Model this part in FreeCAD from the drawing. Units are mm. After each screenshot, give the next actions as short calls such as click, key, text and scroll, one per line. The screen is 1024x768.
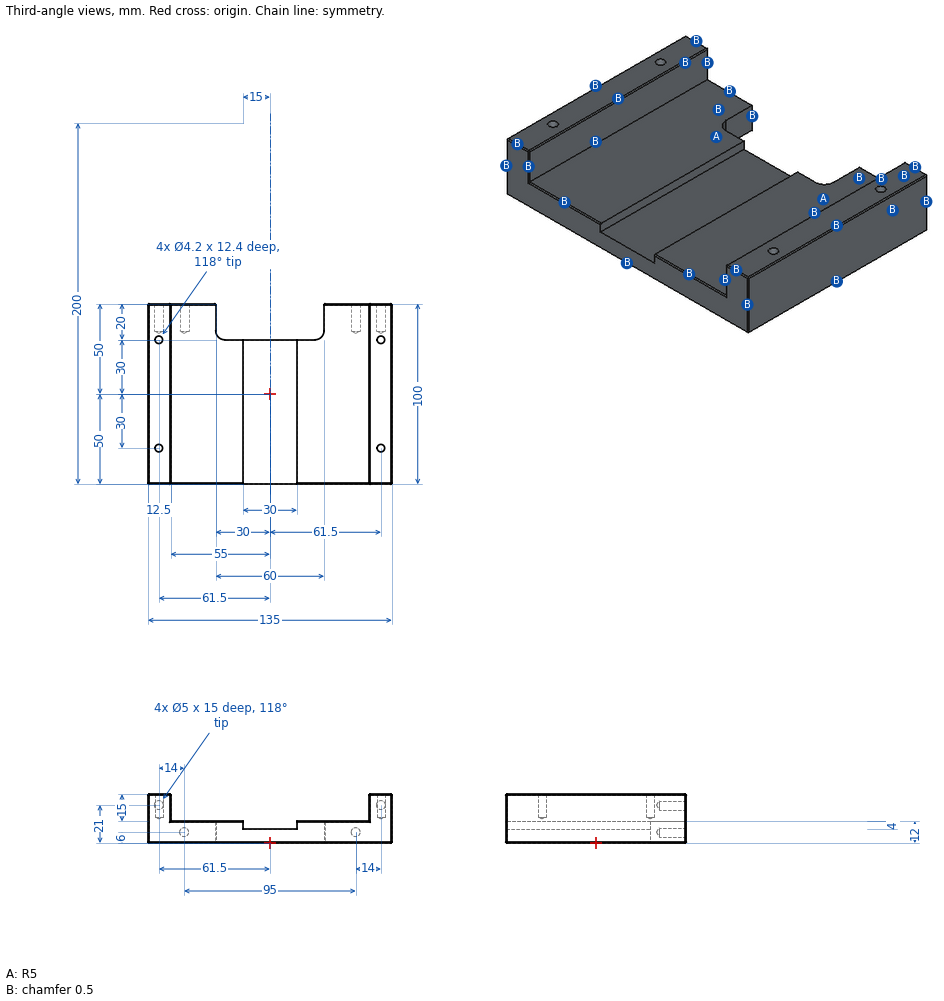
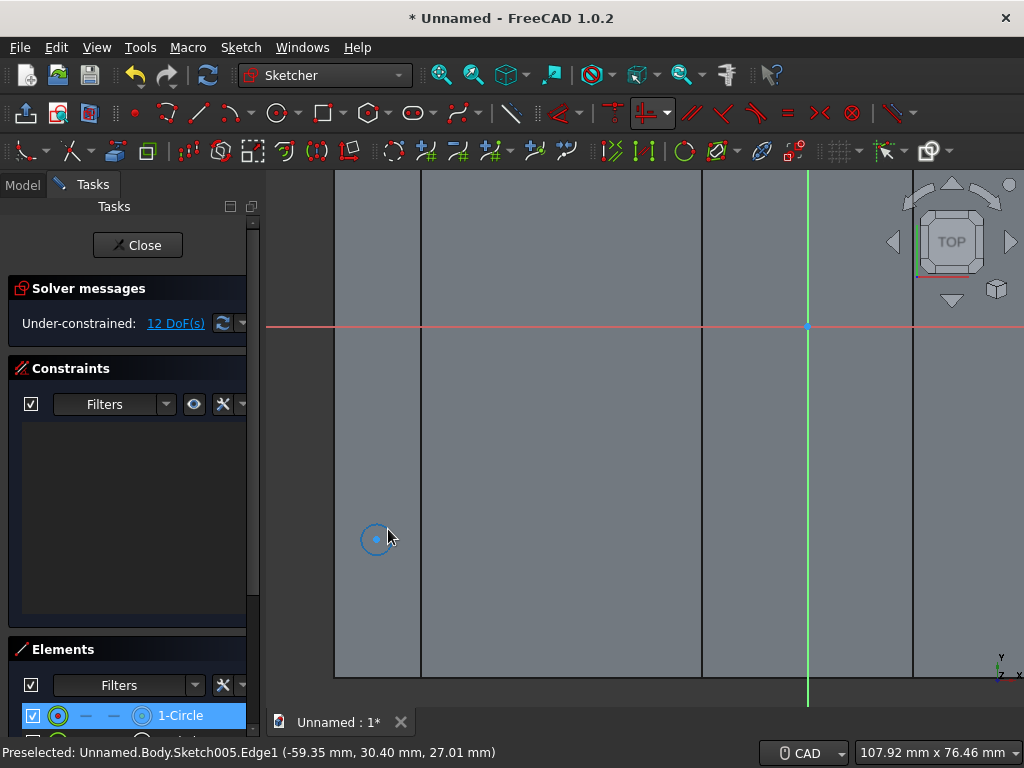
click(388, 529)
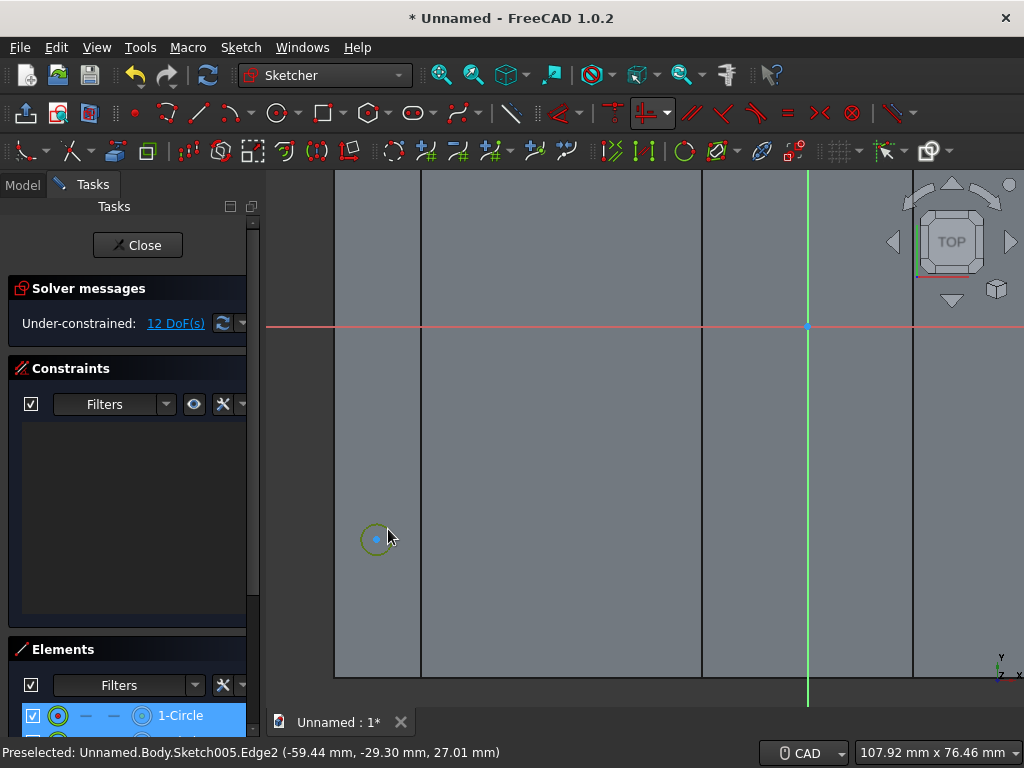
scroll(388, 530, down, 4)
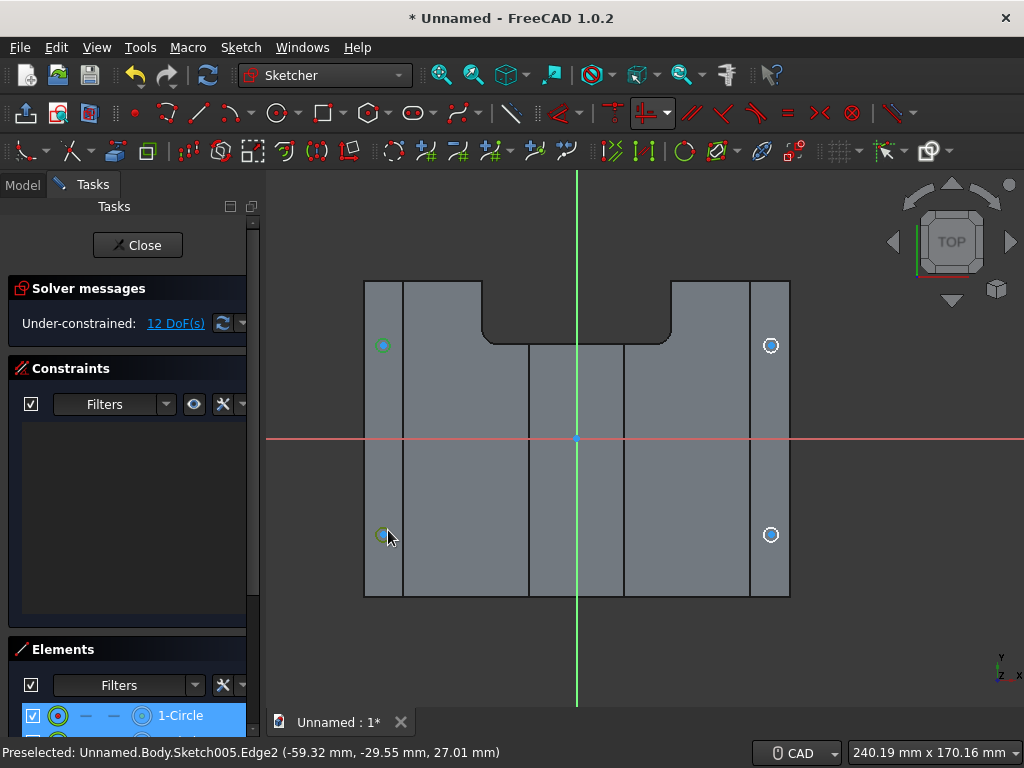
scroll(776, 530, up, 4)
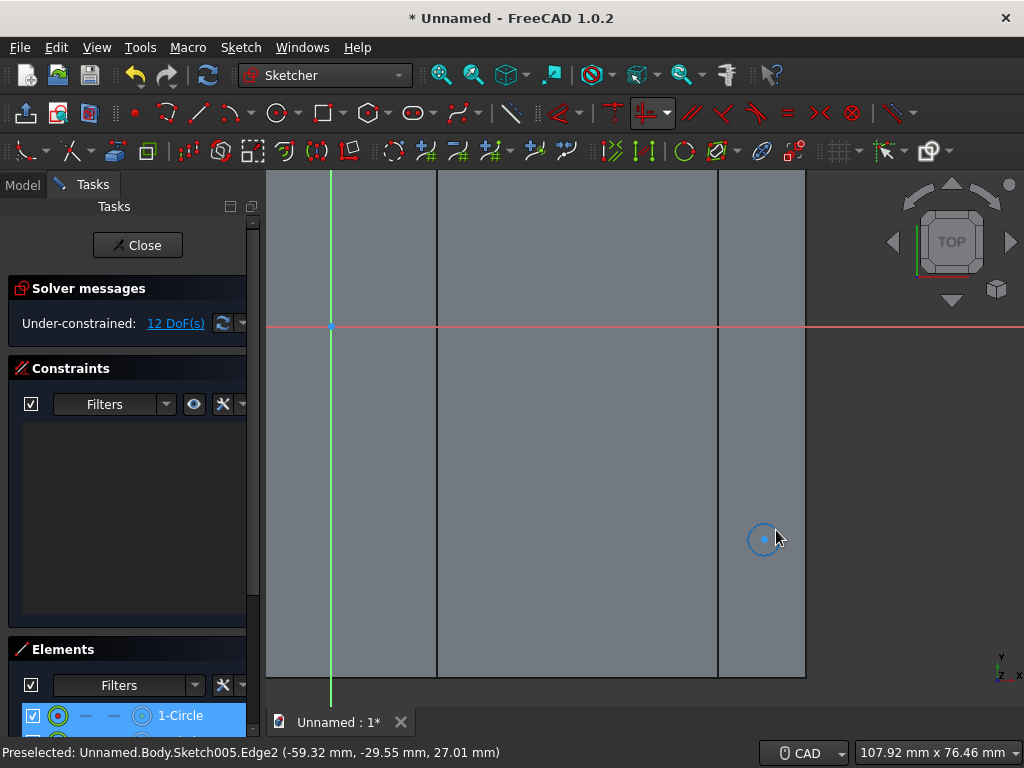
click(775, 529)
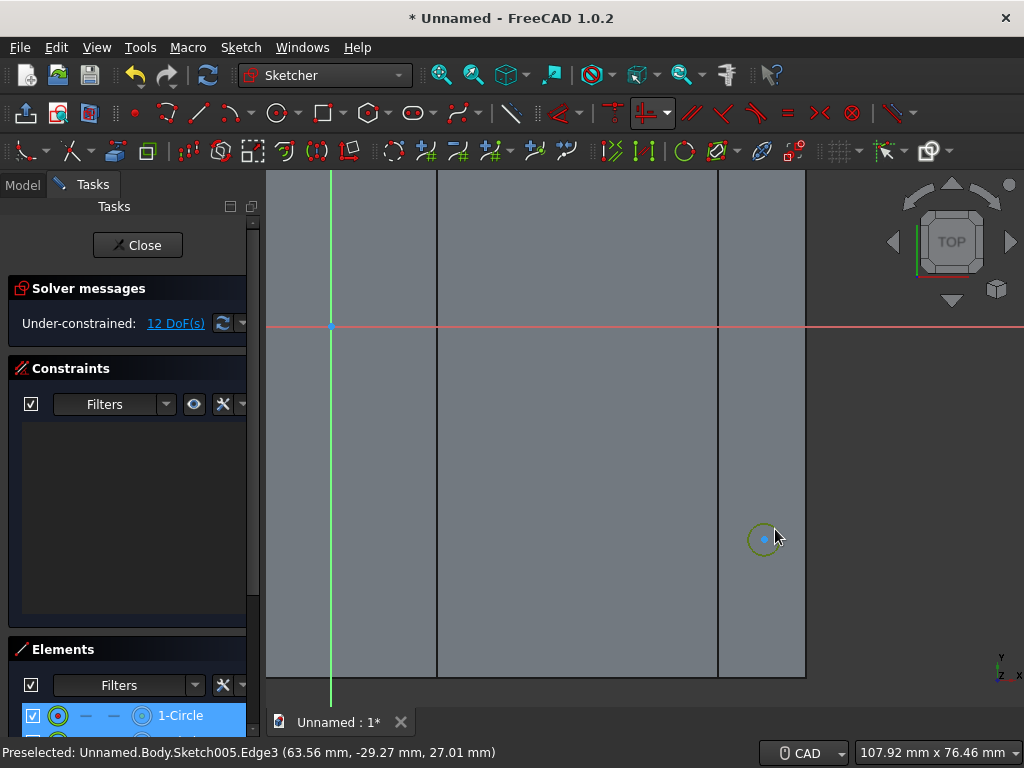
scroll(776, 530, down, 4)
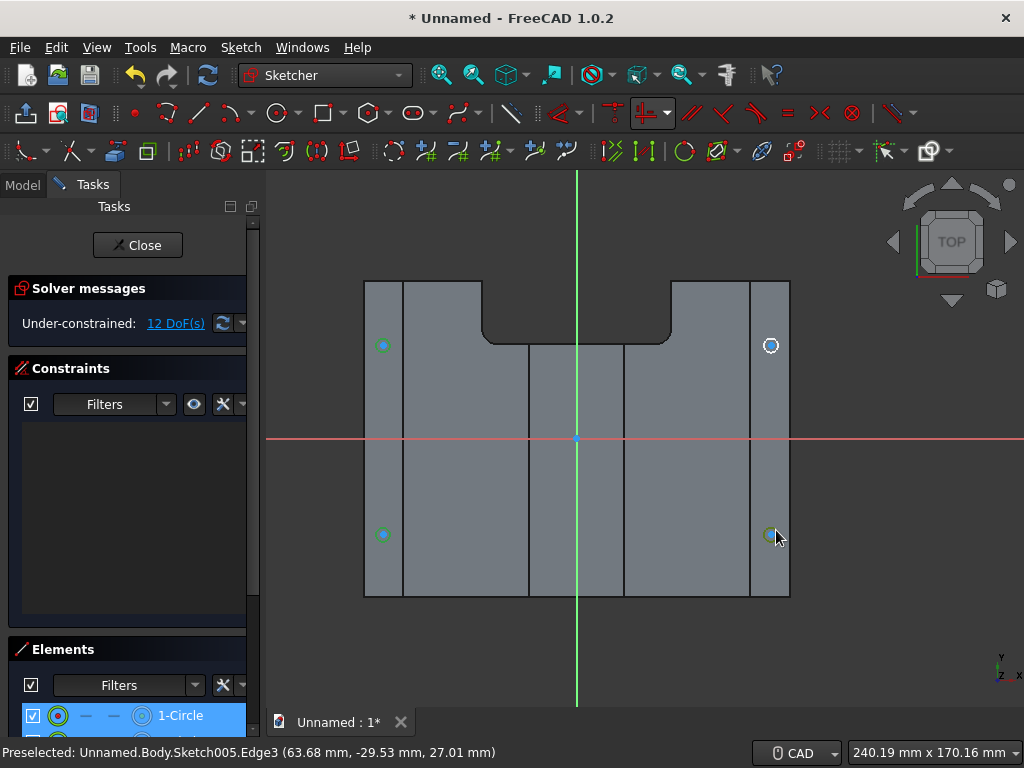
scroll(776, 341, up, 4)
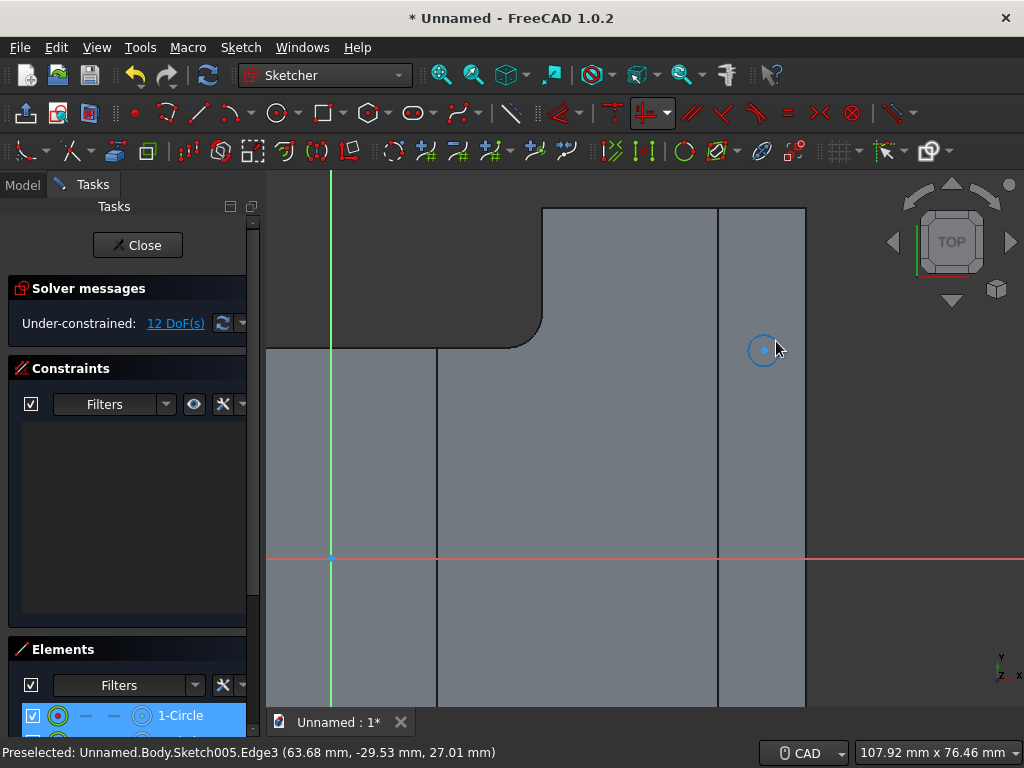
click(775, 340)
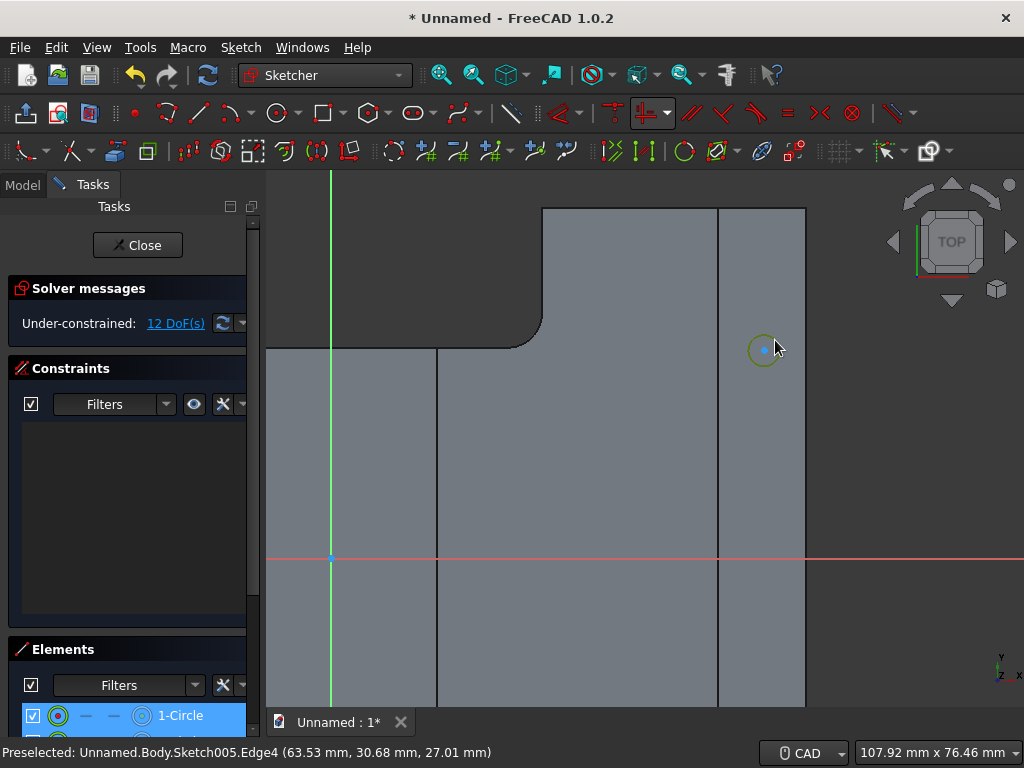
key(e)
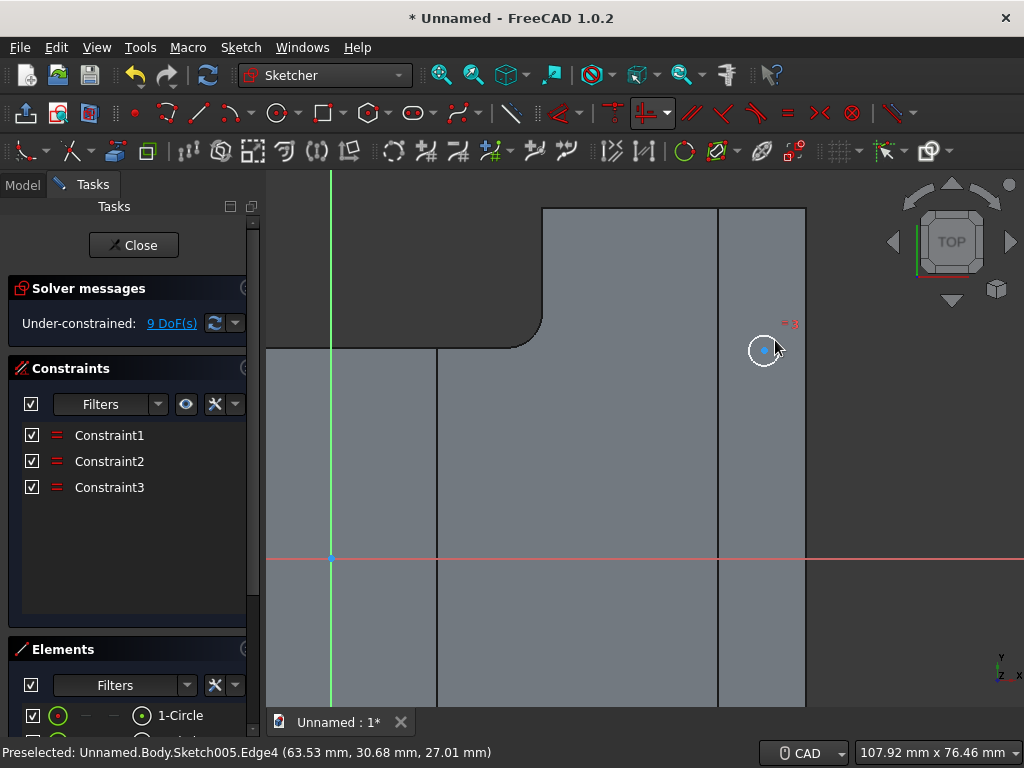
scroll(776, 340, down, 4)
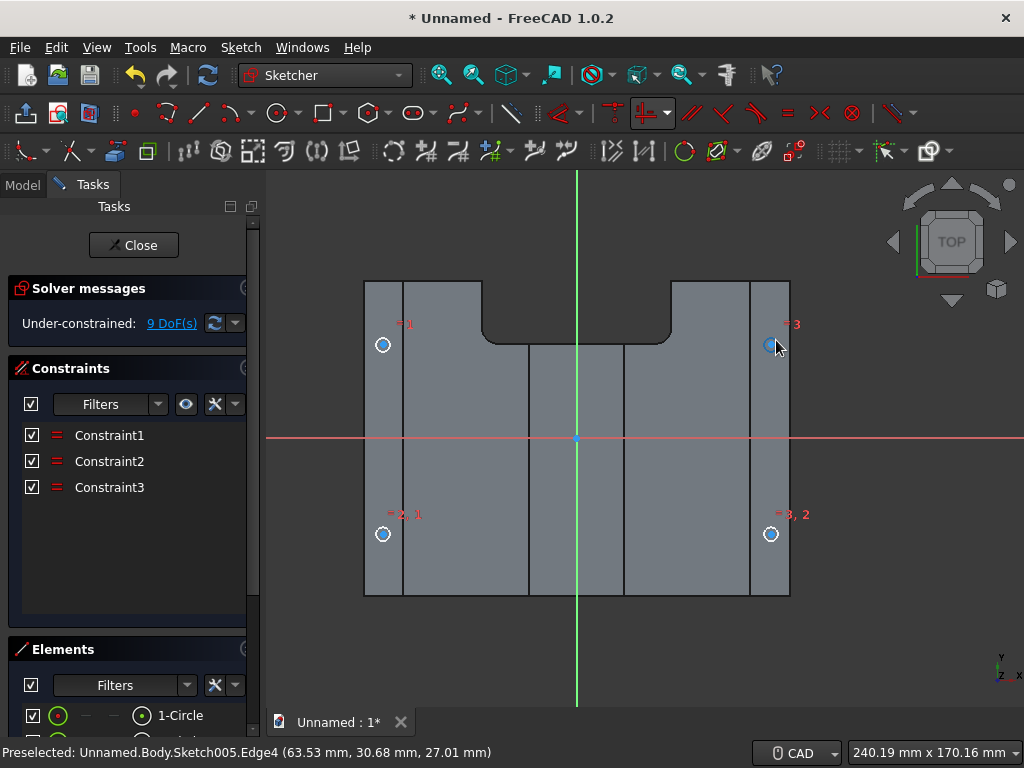
click(383, 345)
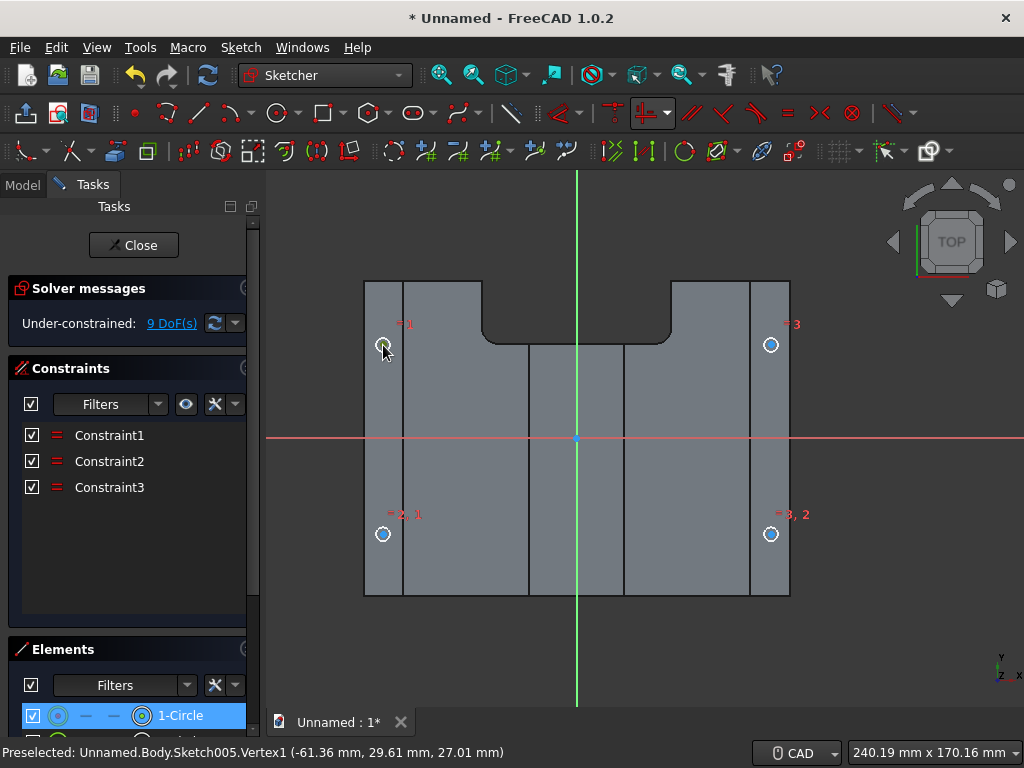
click(383, 534)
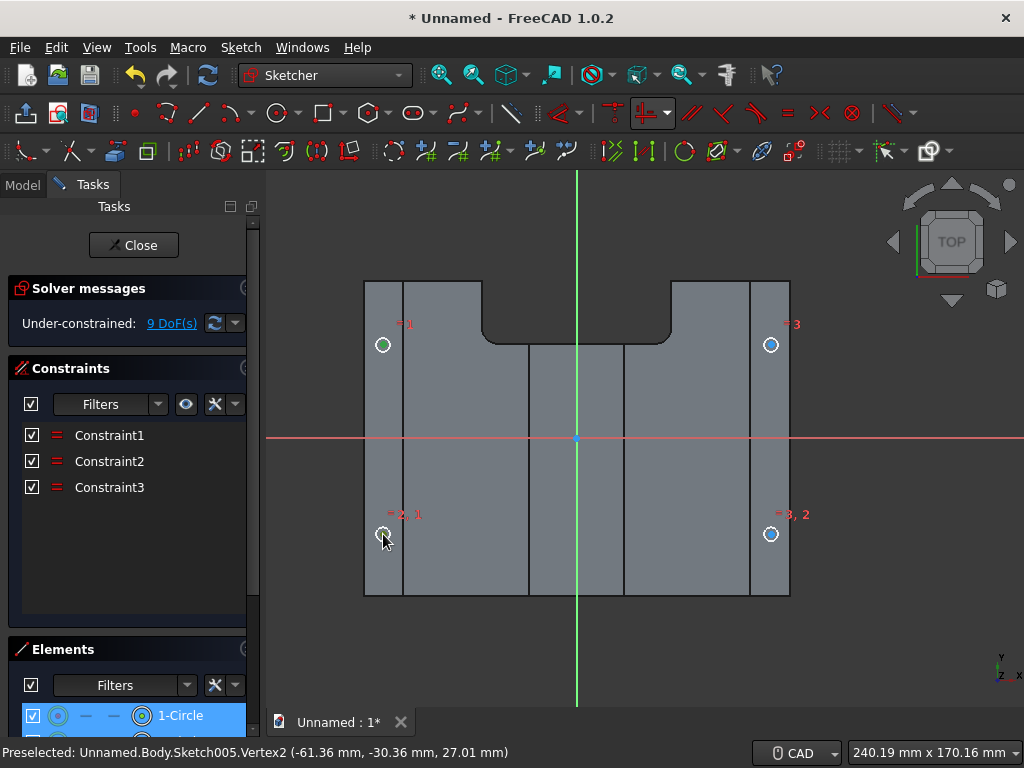
click(670, 114)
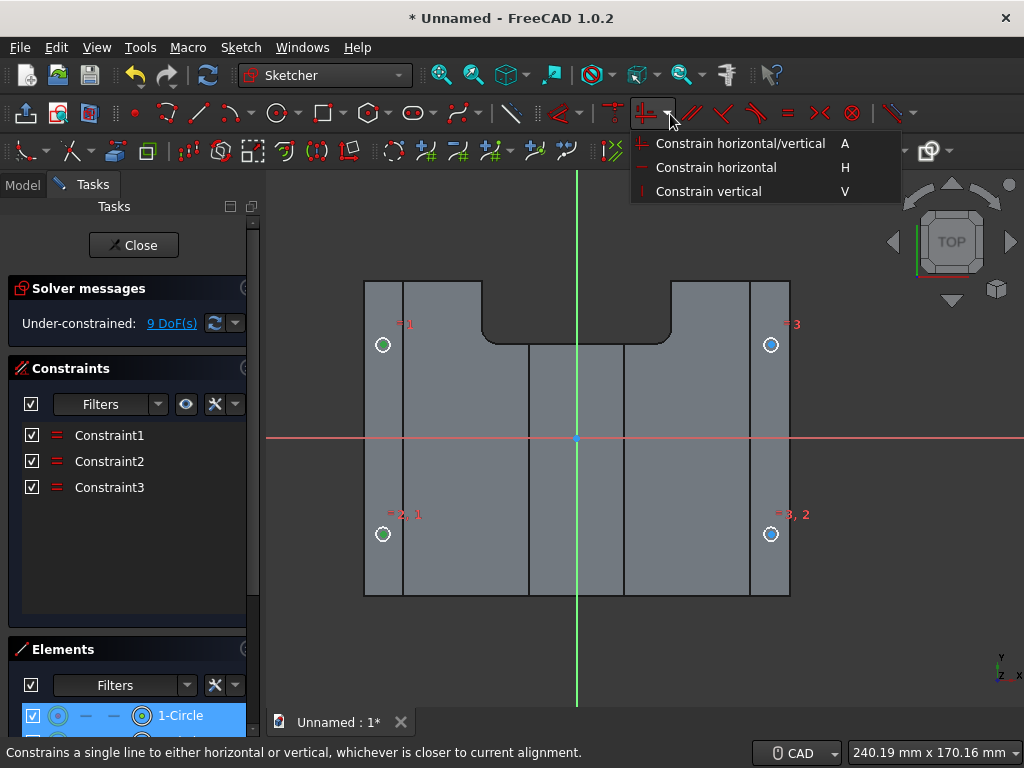
click(766, 191)